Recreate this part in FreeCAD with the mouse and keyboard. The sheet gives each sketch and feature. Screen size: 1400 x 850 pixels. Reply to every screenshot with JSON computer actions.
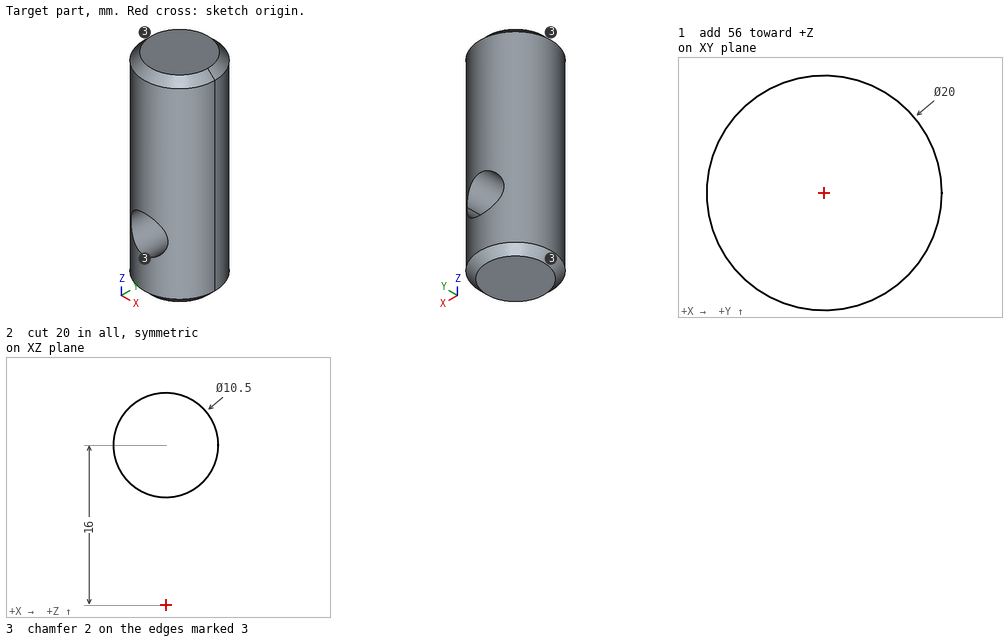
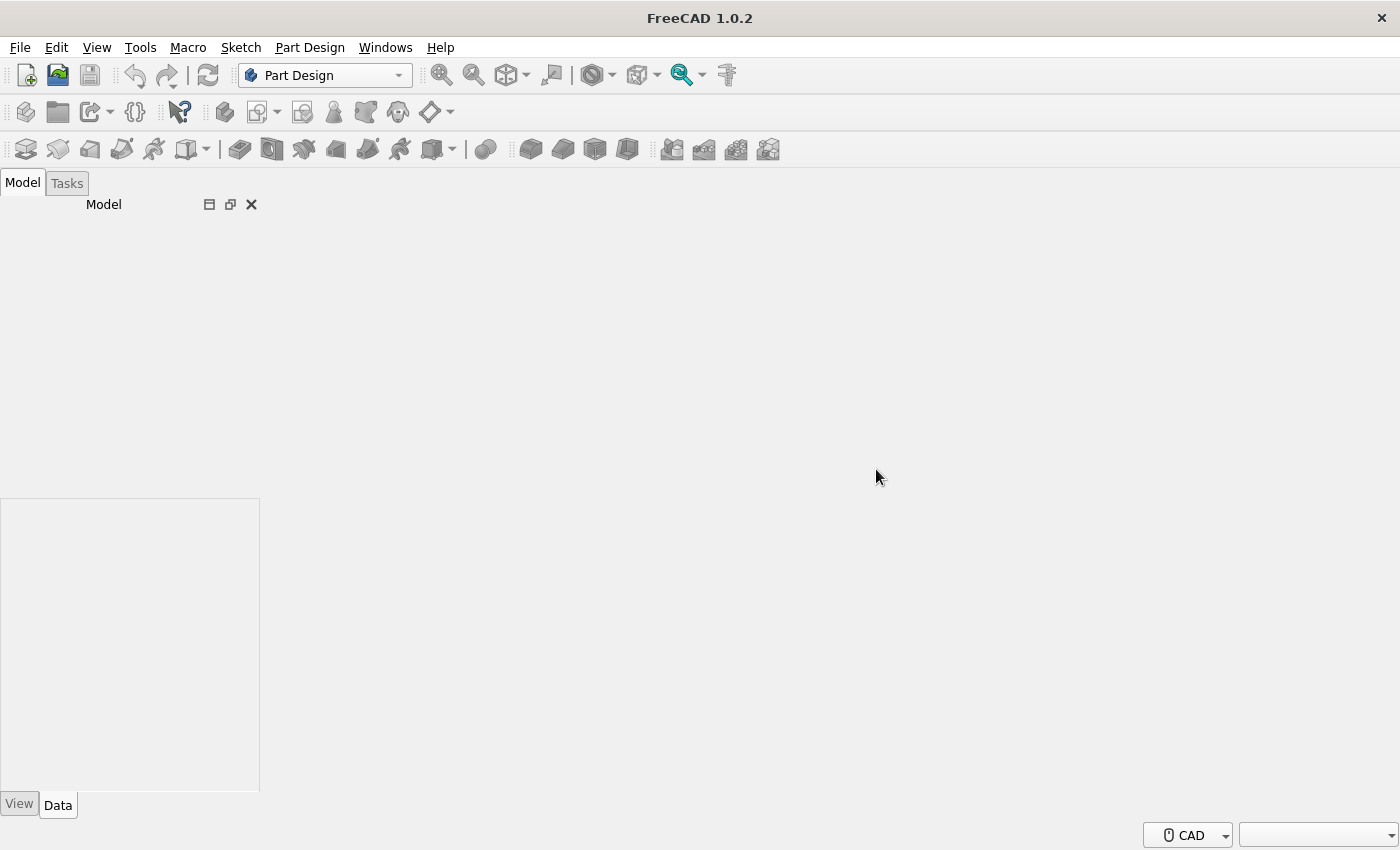
{"action": "left_click", "coordinate": [26, 76]}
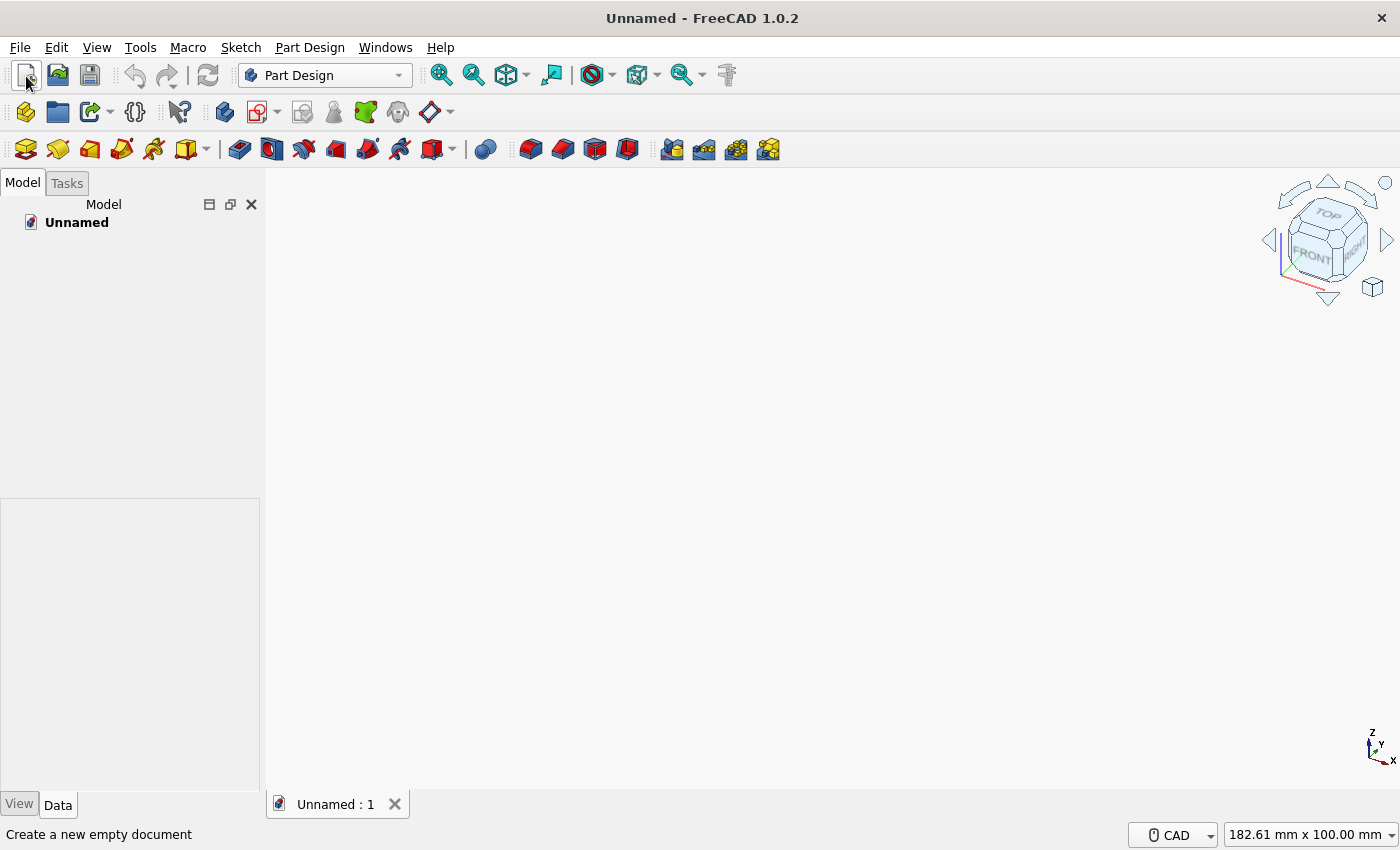
{"action": "left_click", "coordinate": [258, 112]}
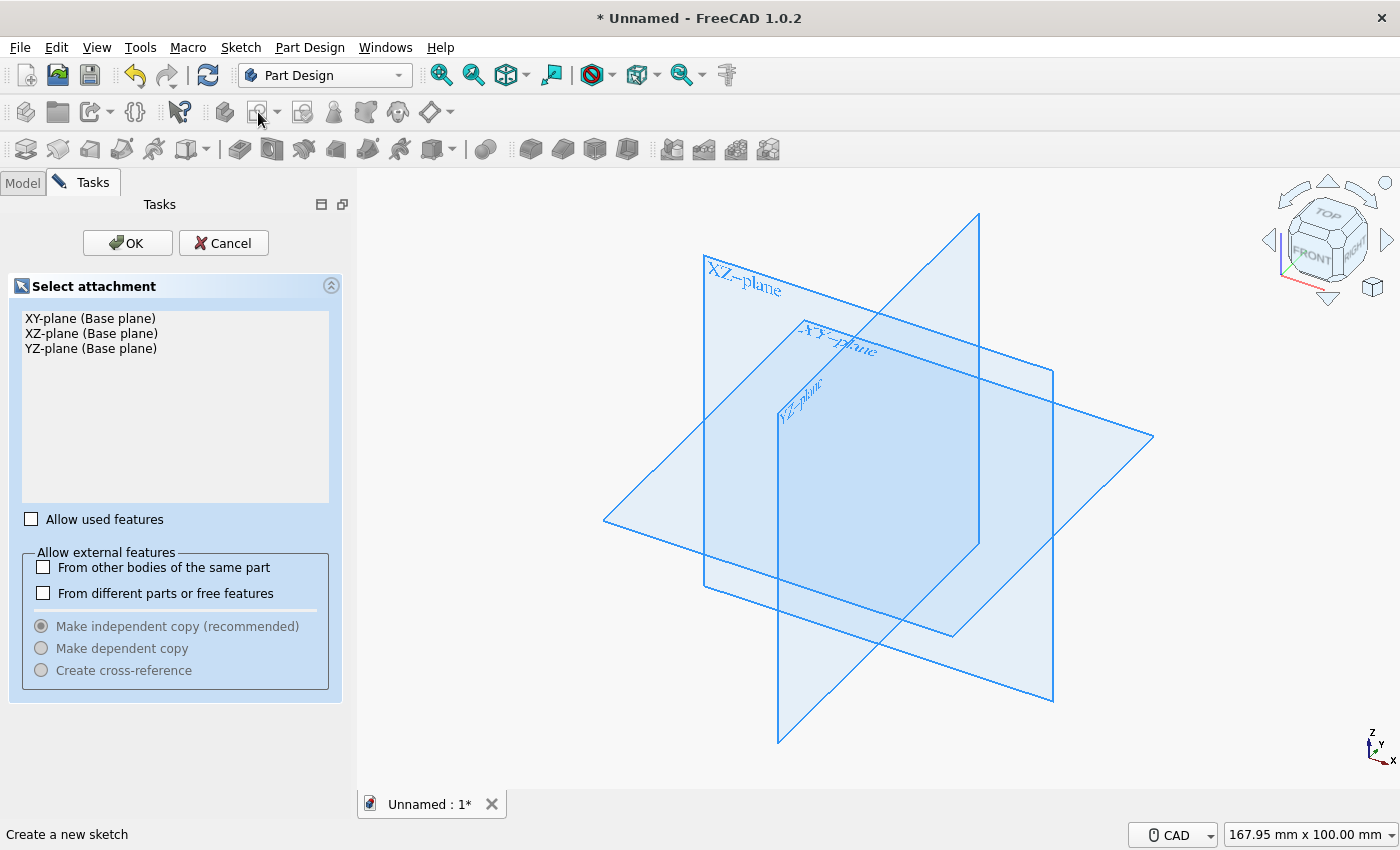
{"action": "left_click", "coordinate": [82, 318]}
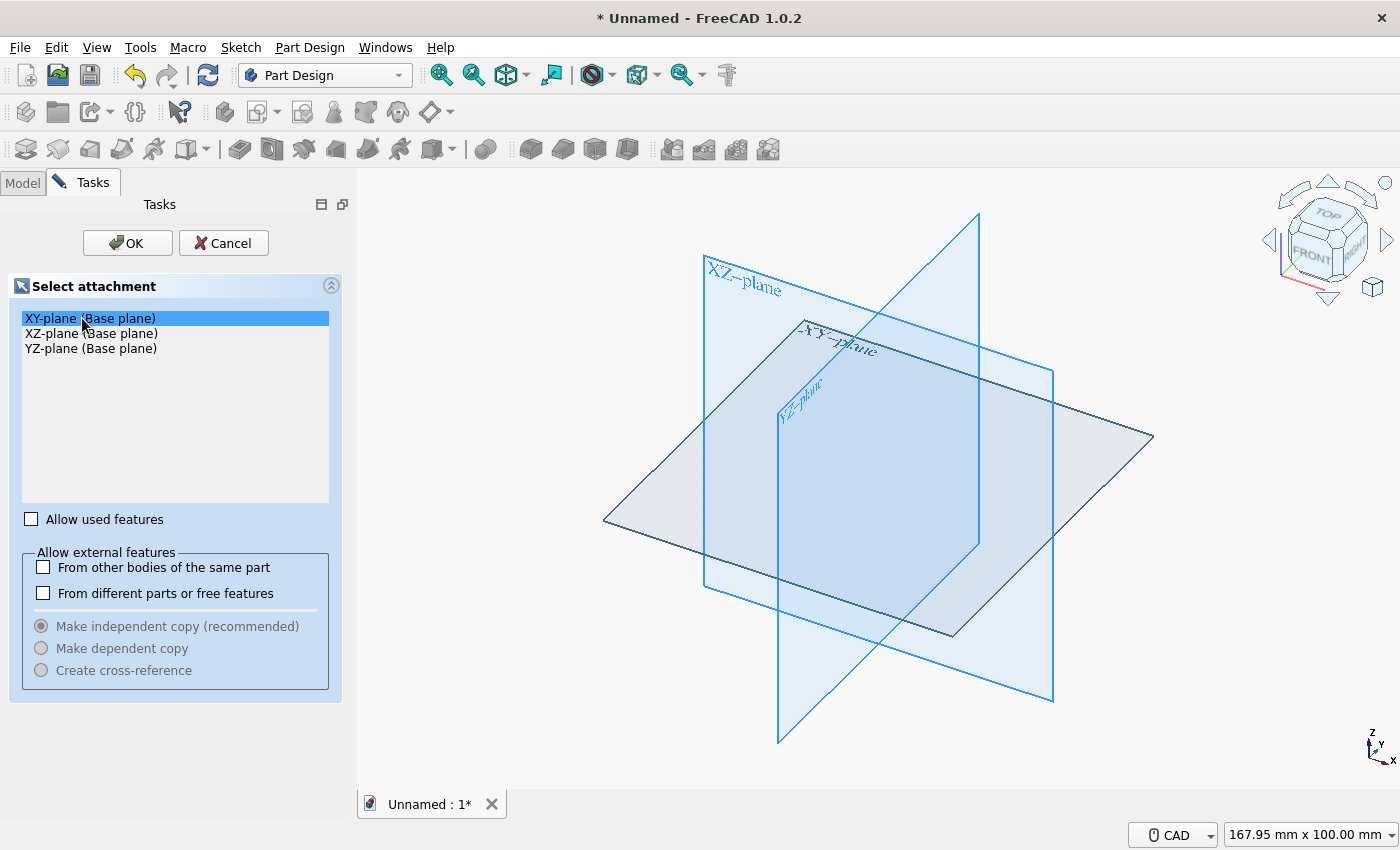
{"action": "left_click", "coordinate": [128, 243]}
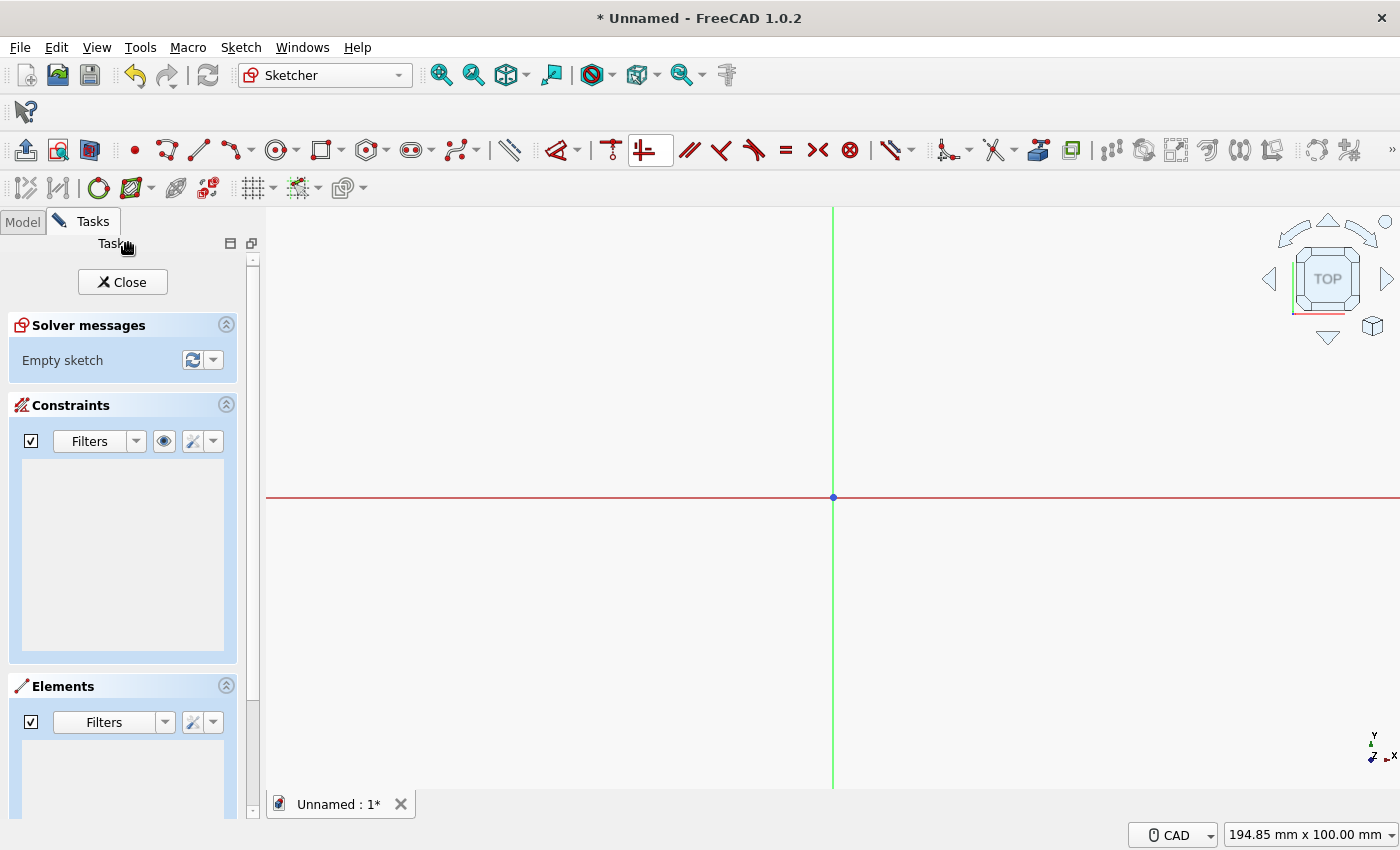
{"action": "scroll", "coordinate": [863, 498], "scroll_direction": "up", "scroll_amount": 6}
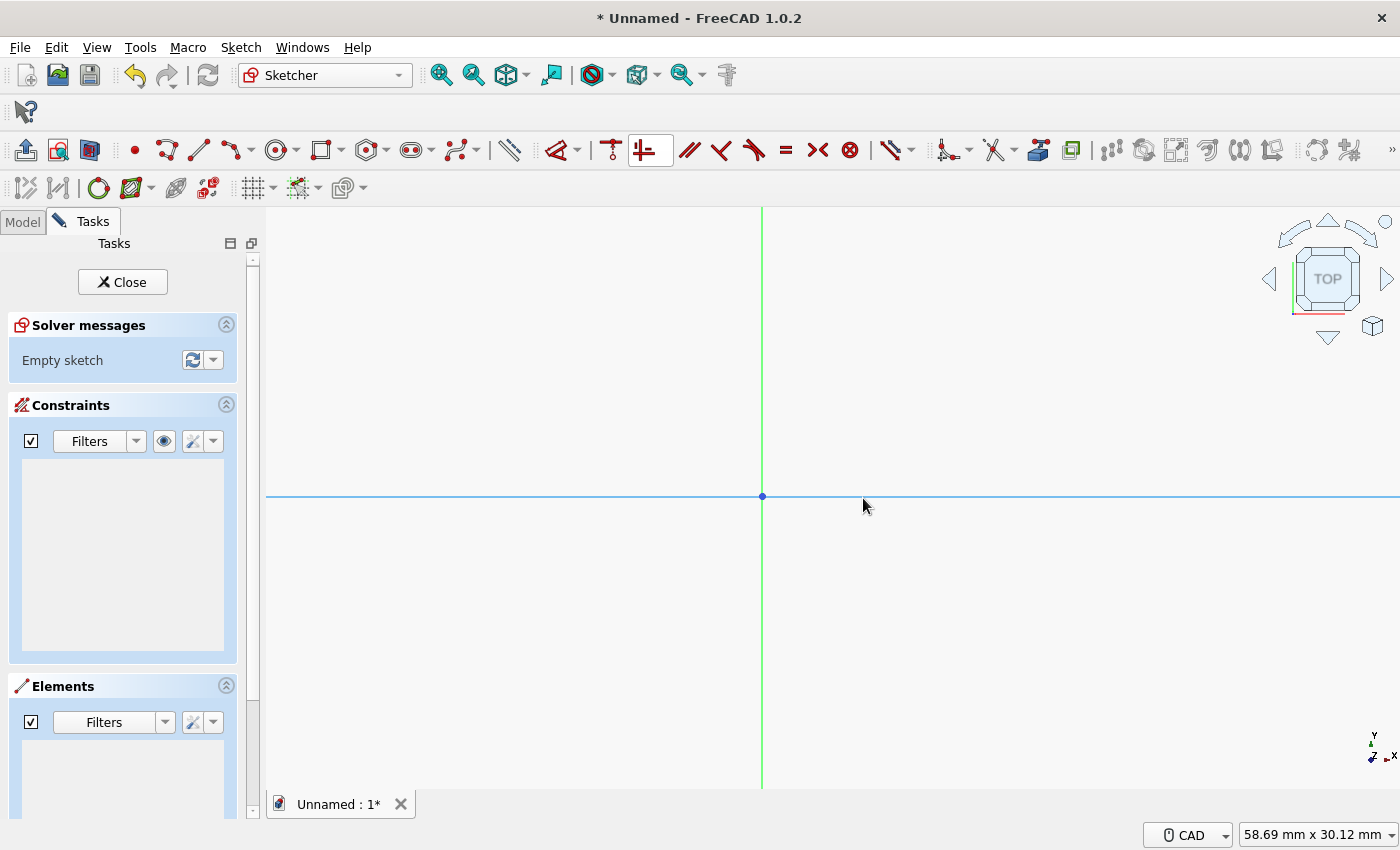
{"action": "left_click", "coordinate": [276, 150]}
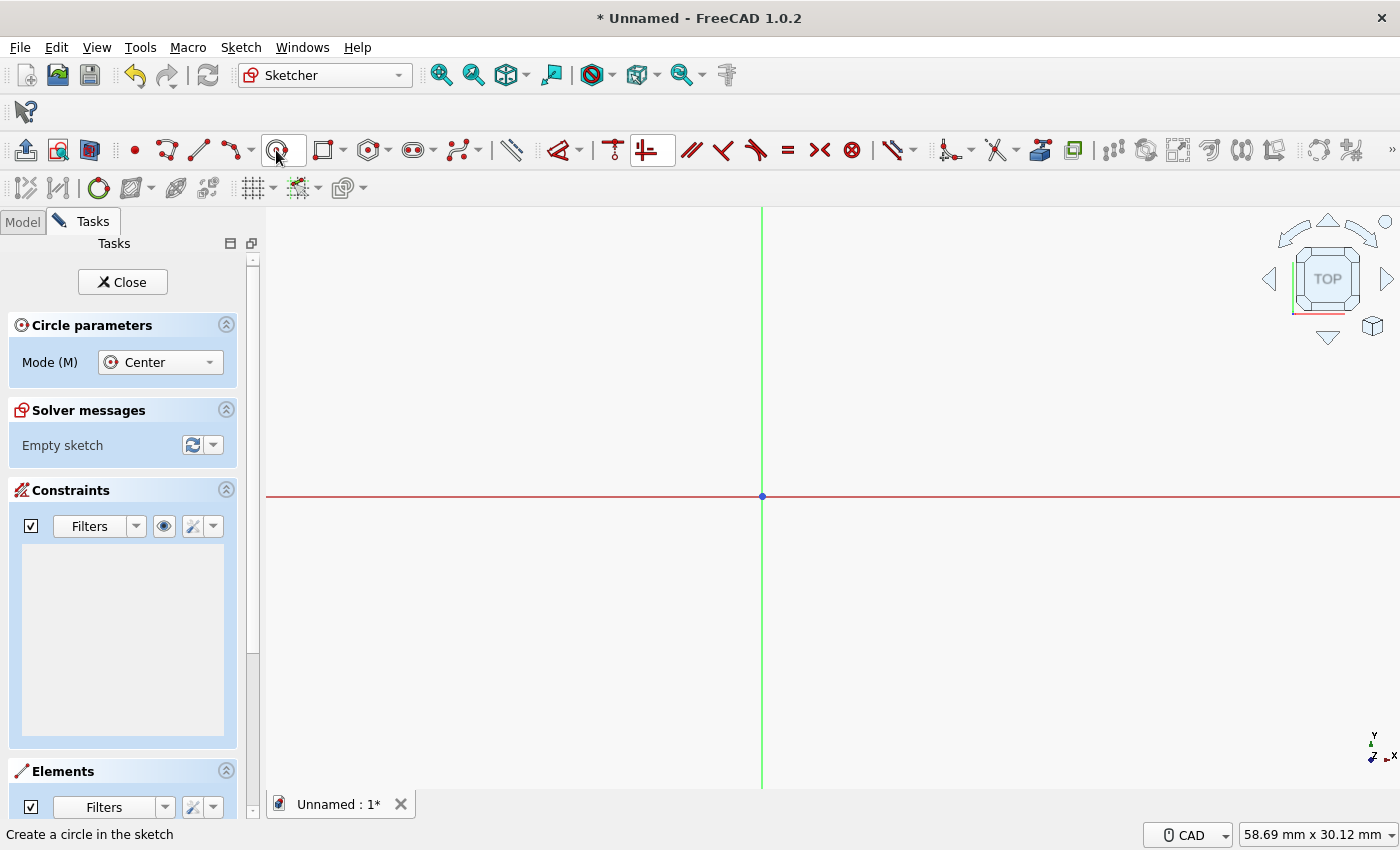
{"action": "left_click", "coordinate": [762, 497]}
{"action": "left_click", "coordinate": [899, 360]}
{"action": "key", "text": "Escape"}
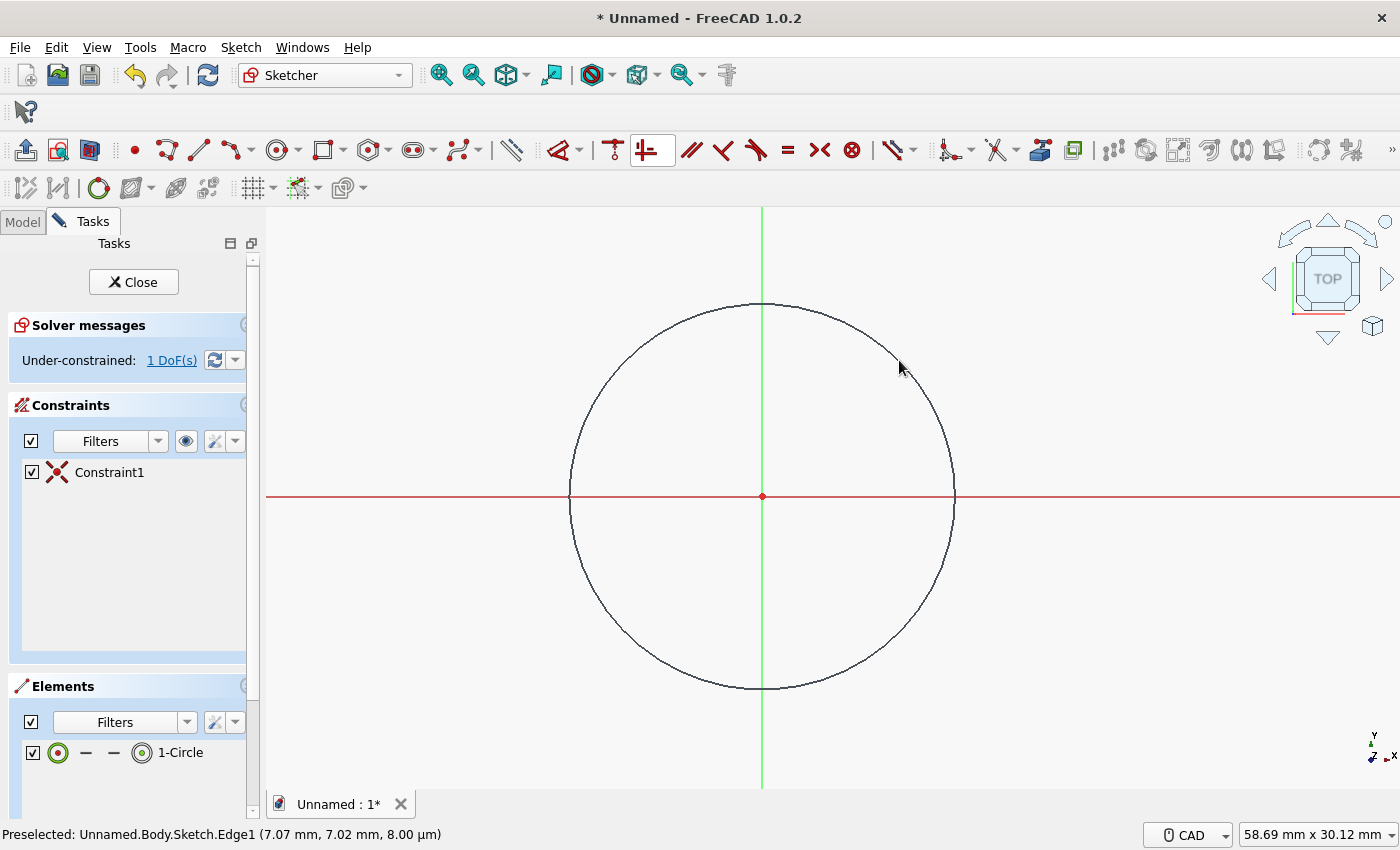
{"action": "left_click", "coordinate": [558, 150]}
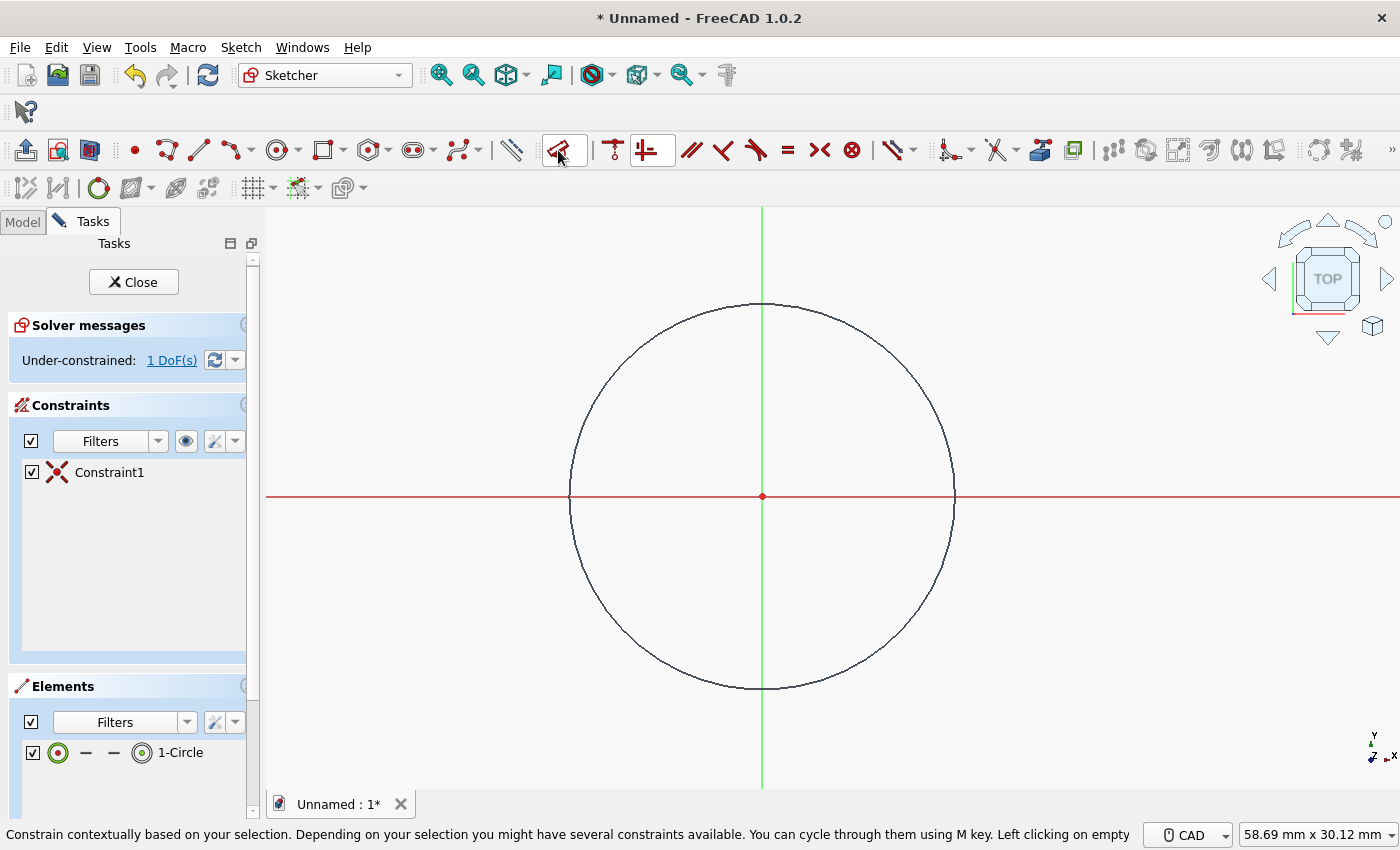
{"action": "left_click", "coordinate": [898, 360]}
{"action": "left_click", "coordinate": [921, 337]}